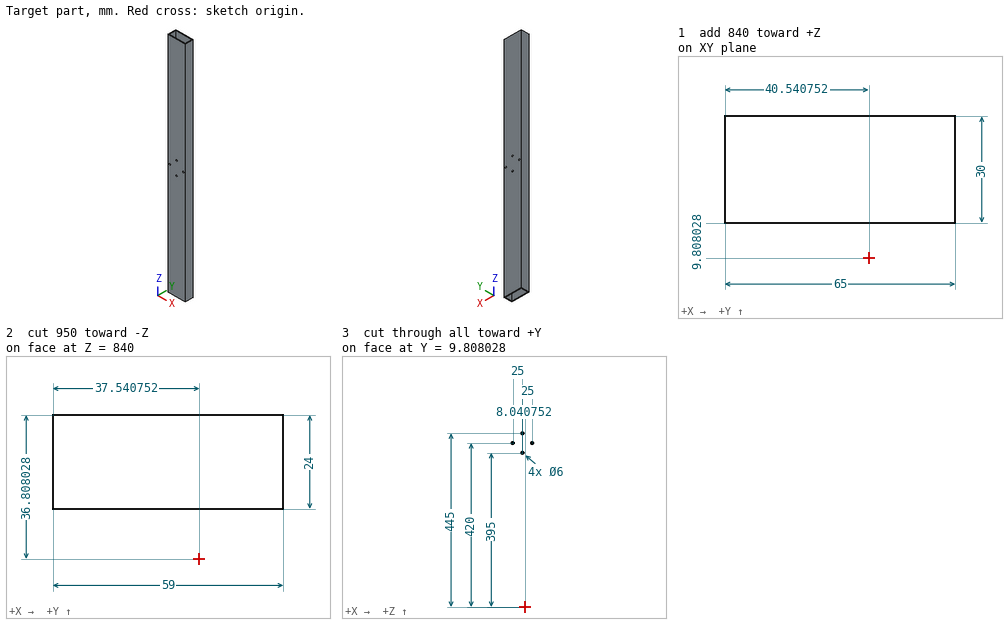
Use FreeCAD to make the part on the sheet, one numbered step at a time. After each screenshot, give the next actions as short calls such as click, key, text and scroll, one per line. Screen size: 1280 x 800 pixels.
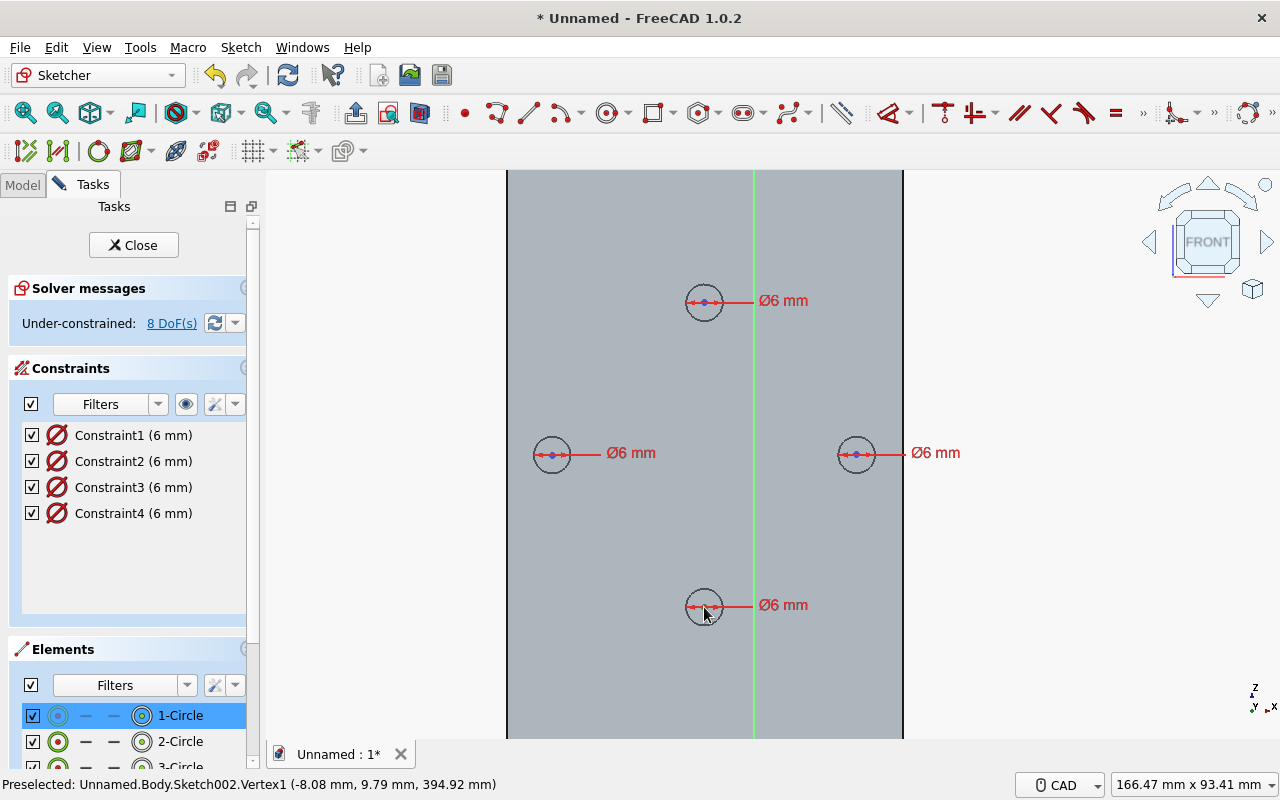
click(704, 303)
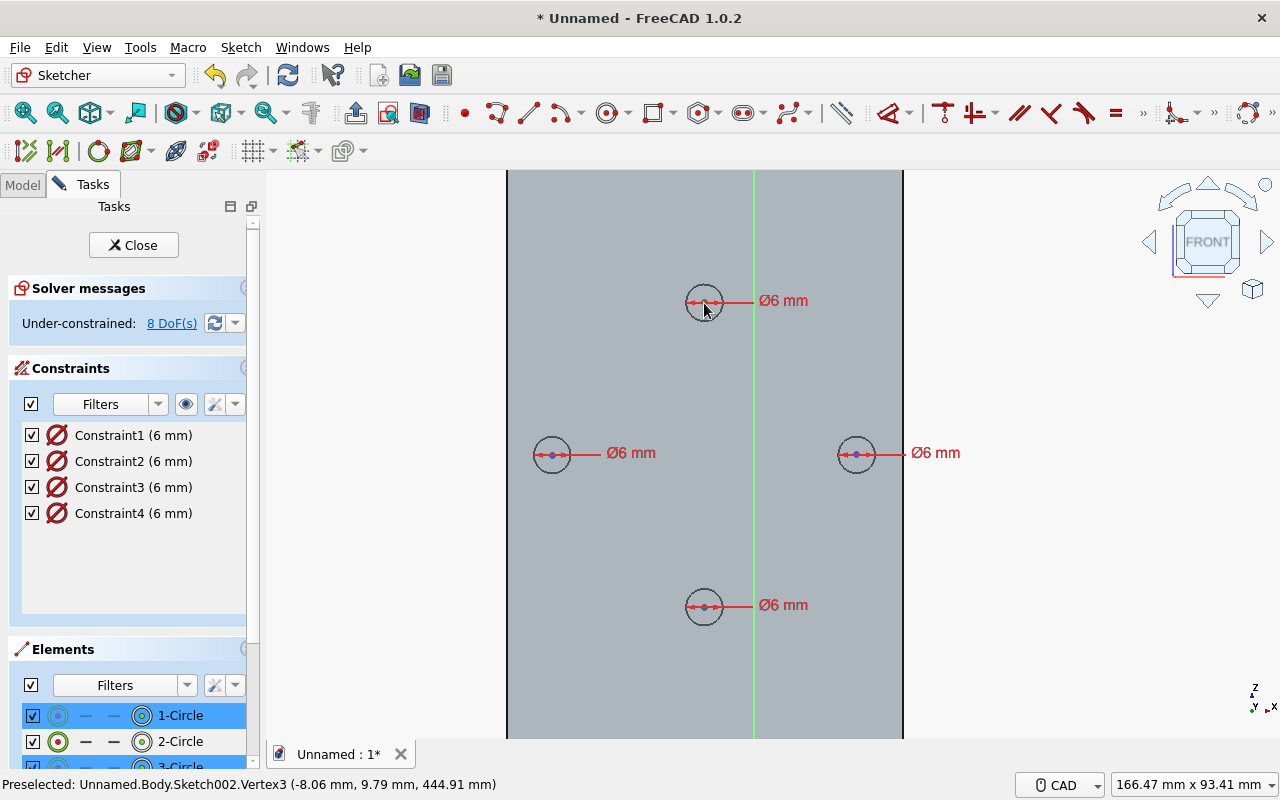
click(998, 114)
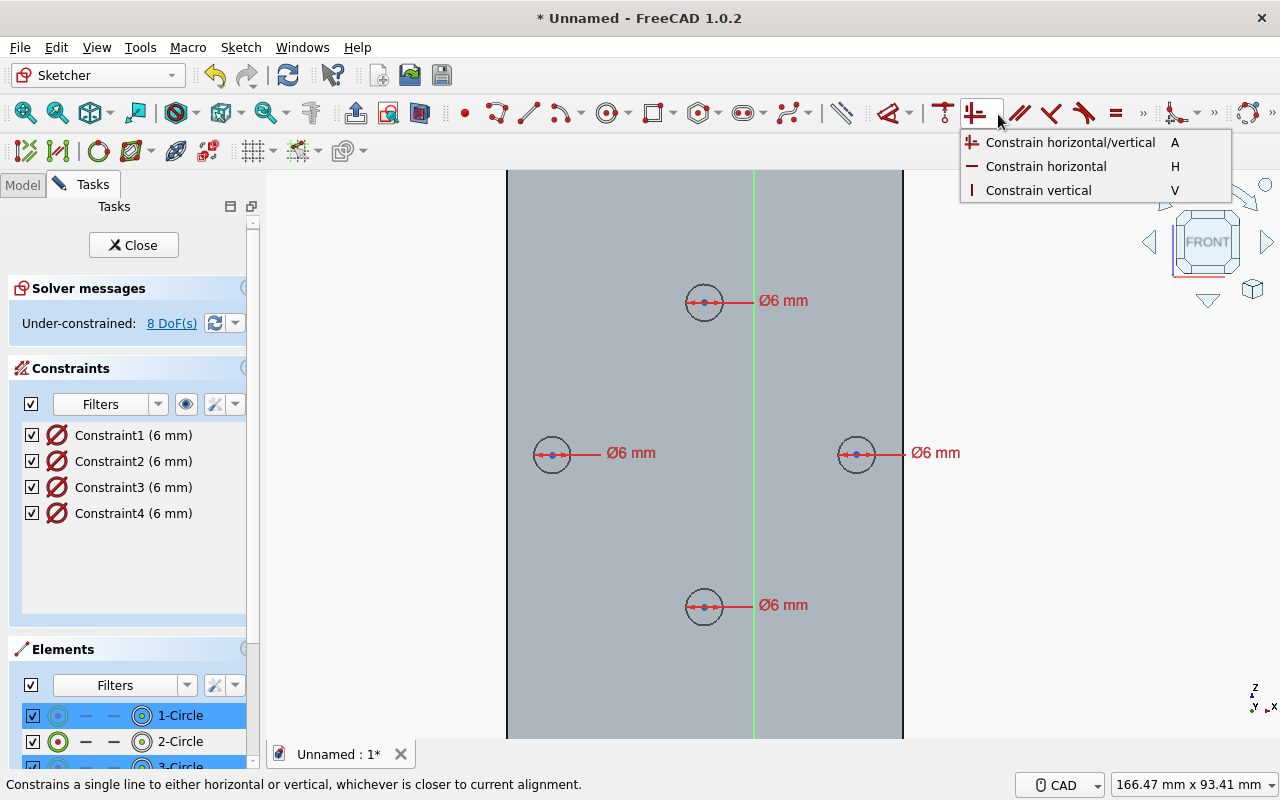
click(1096, 190)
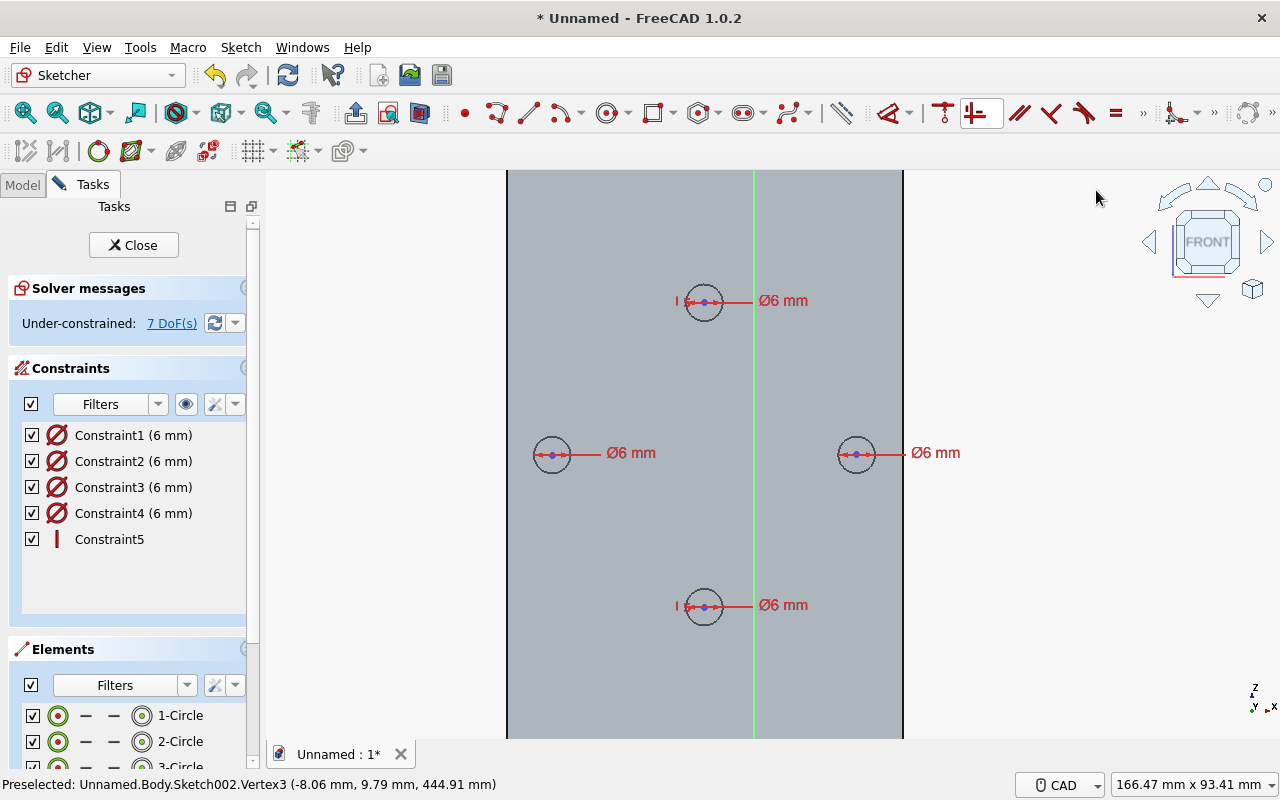
click(552, 455)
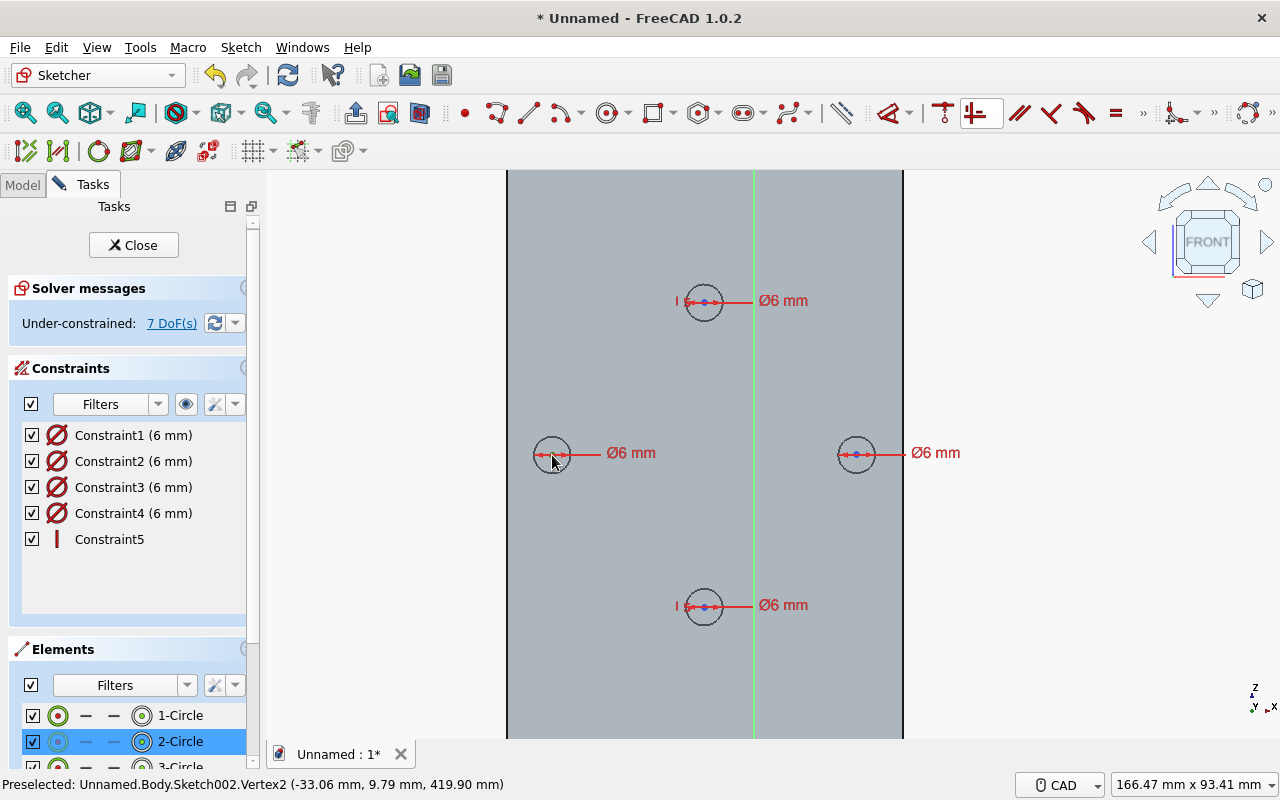
click(857, 455)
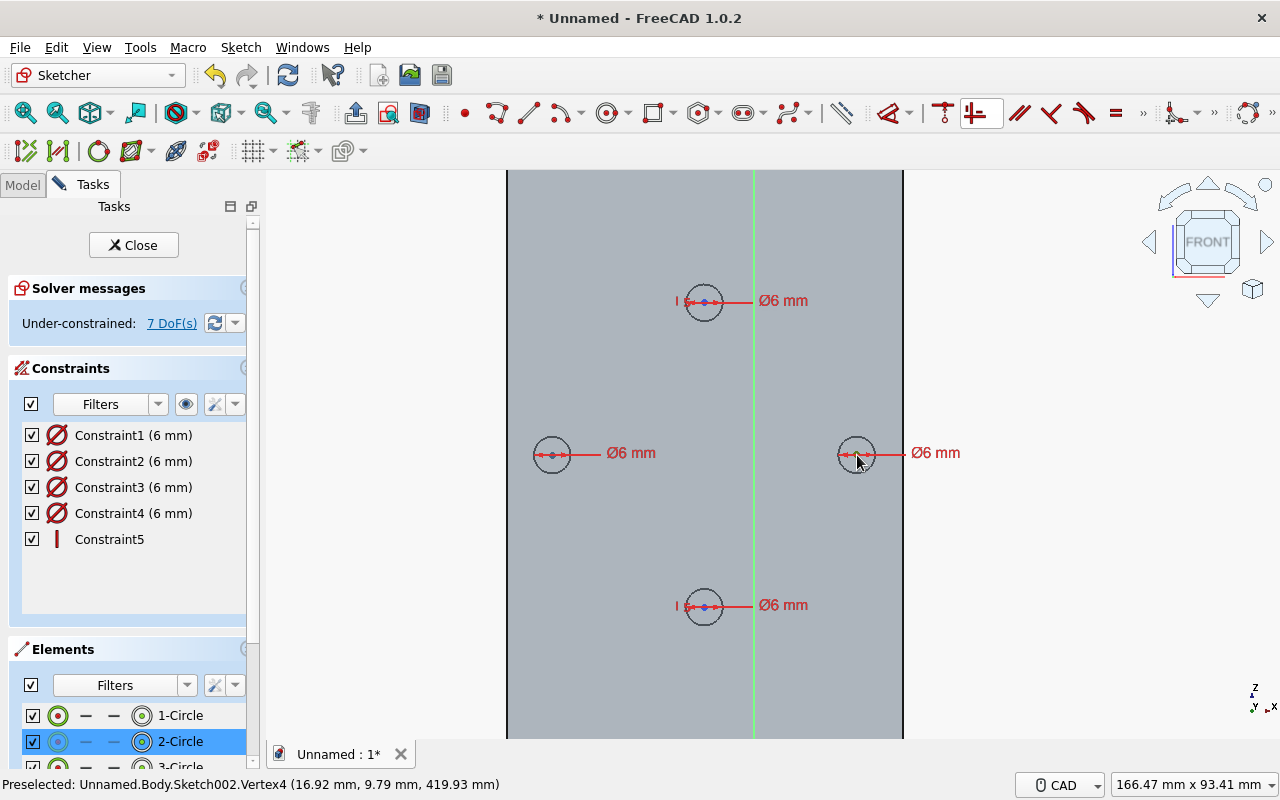
key(h)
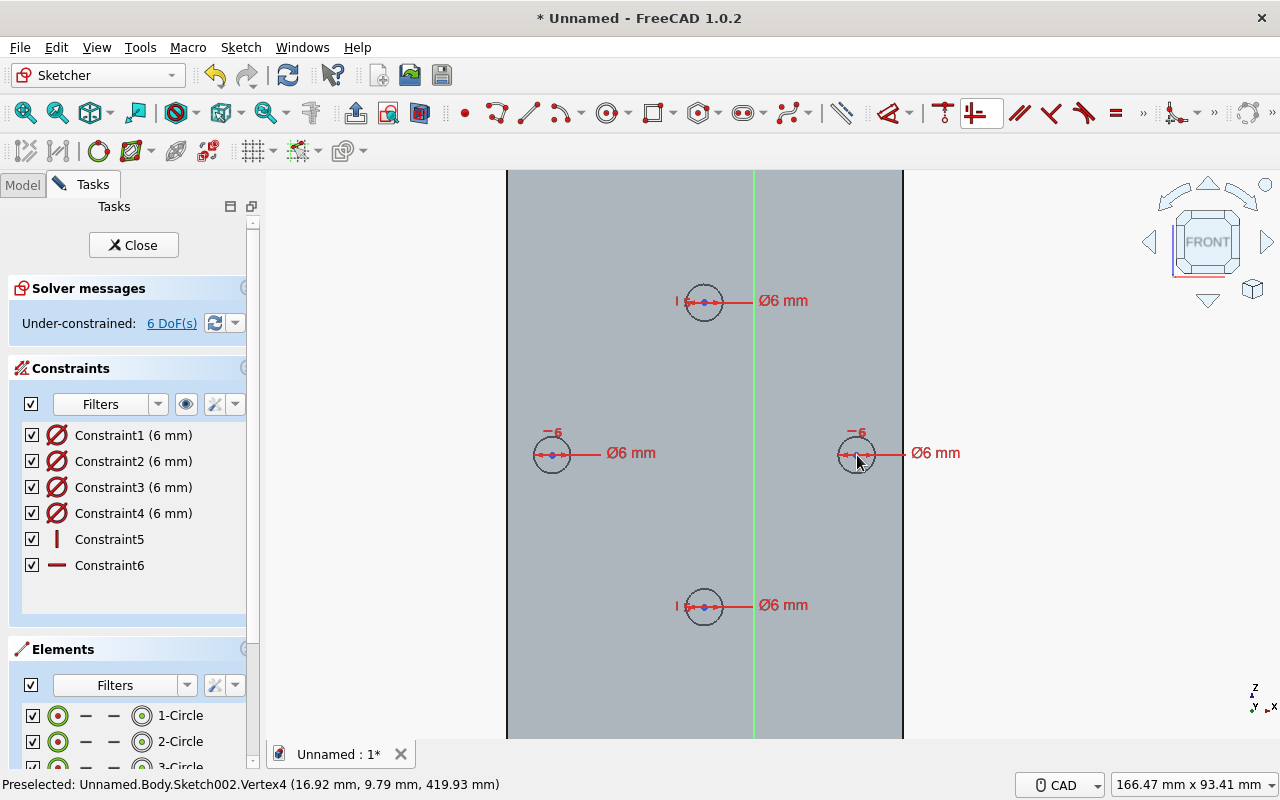
click(888, 114)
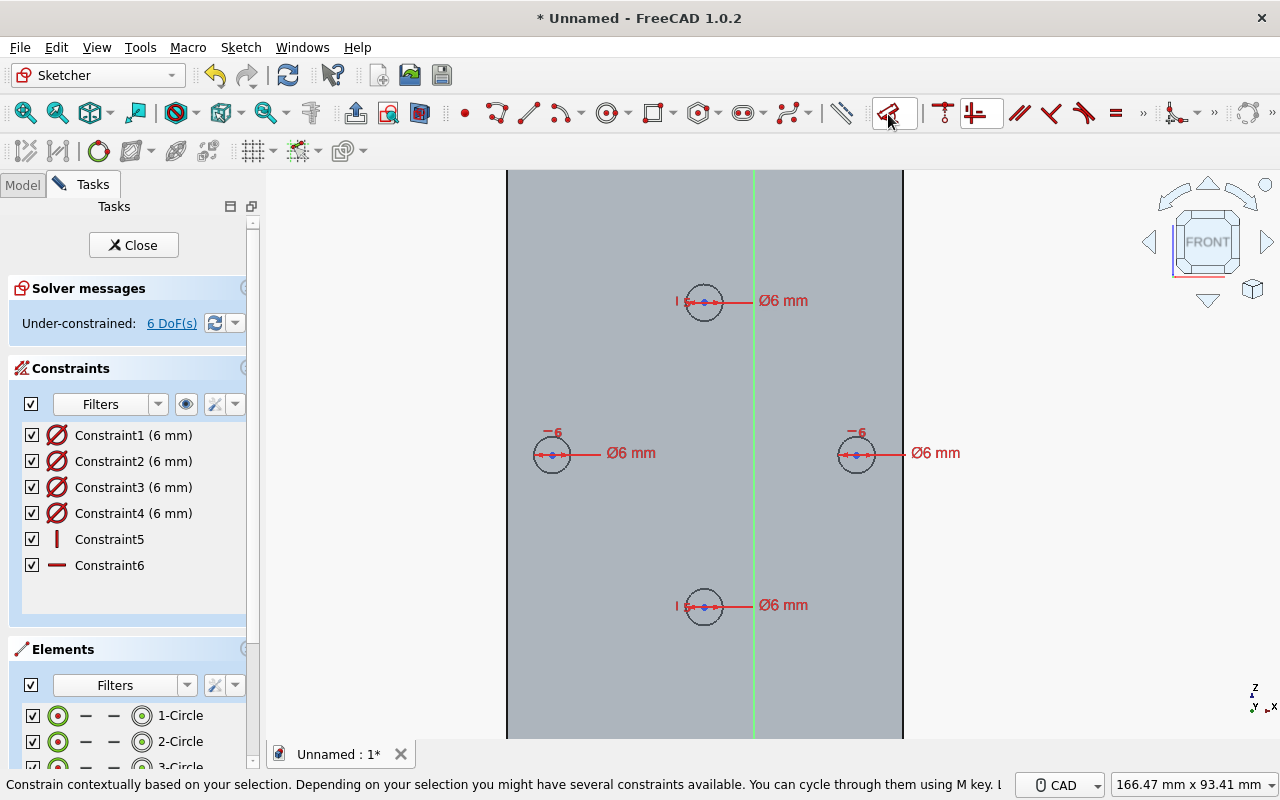
click(704, 607)
click(788, 659)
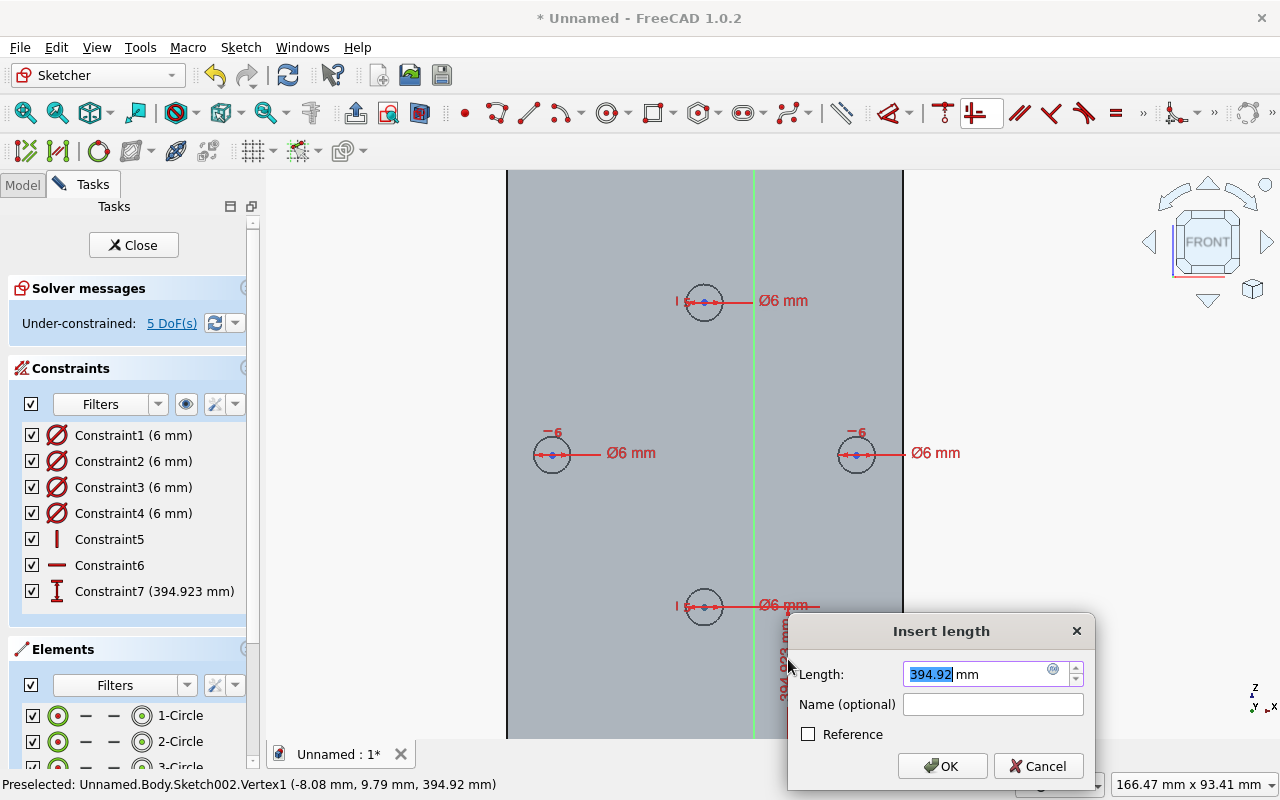
text(395)
key(Return)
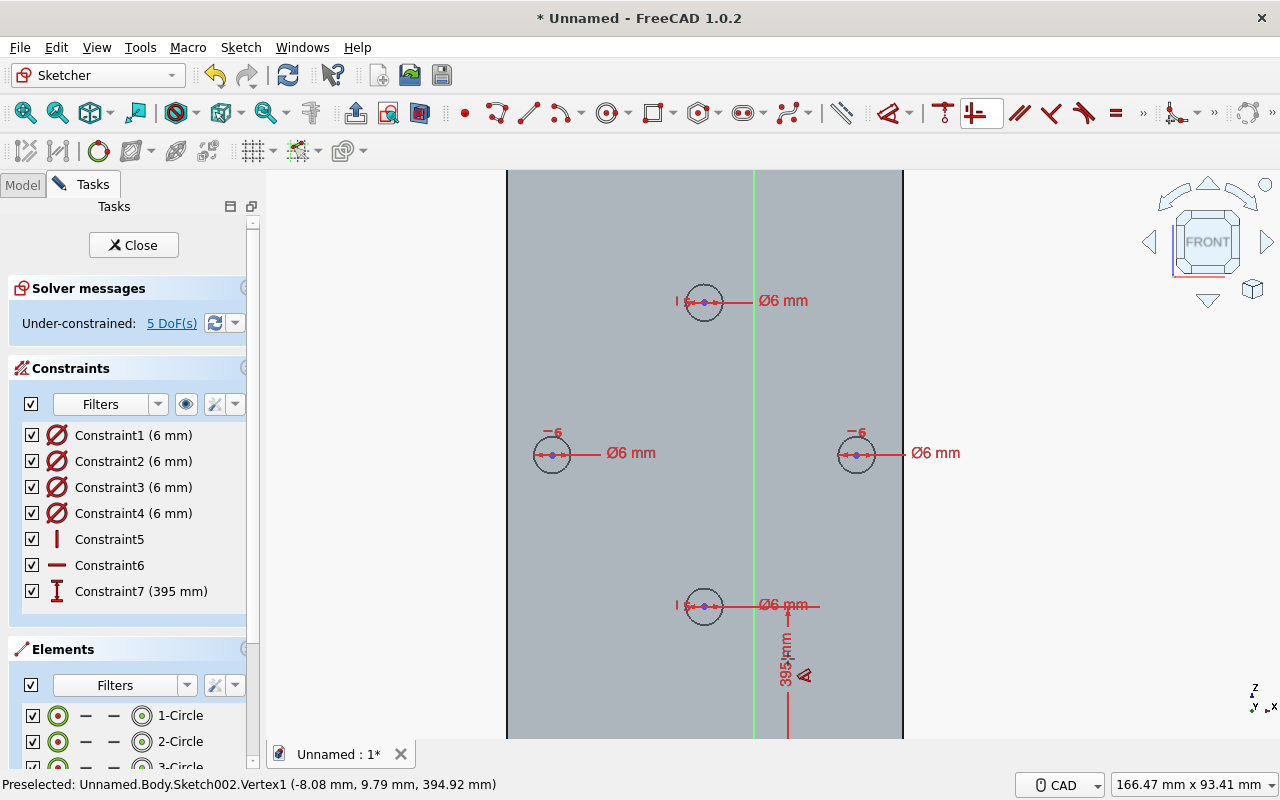
click(552, 455)
click(518, 583)